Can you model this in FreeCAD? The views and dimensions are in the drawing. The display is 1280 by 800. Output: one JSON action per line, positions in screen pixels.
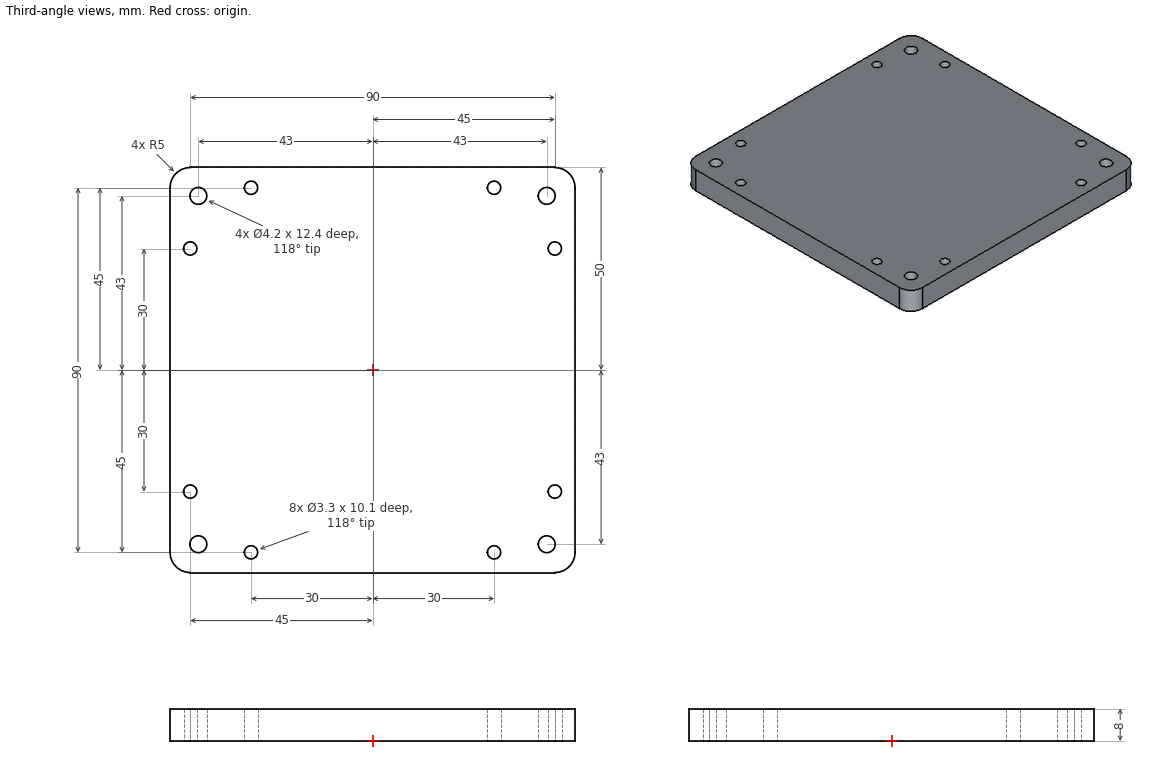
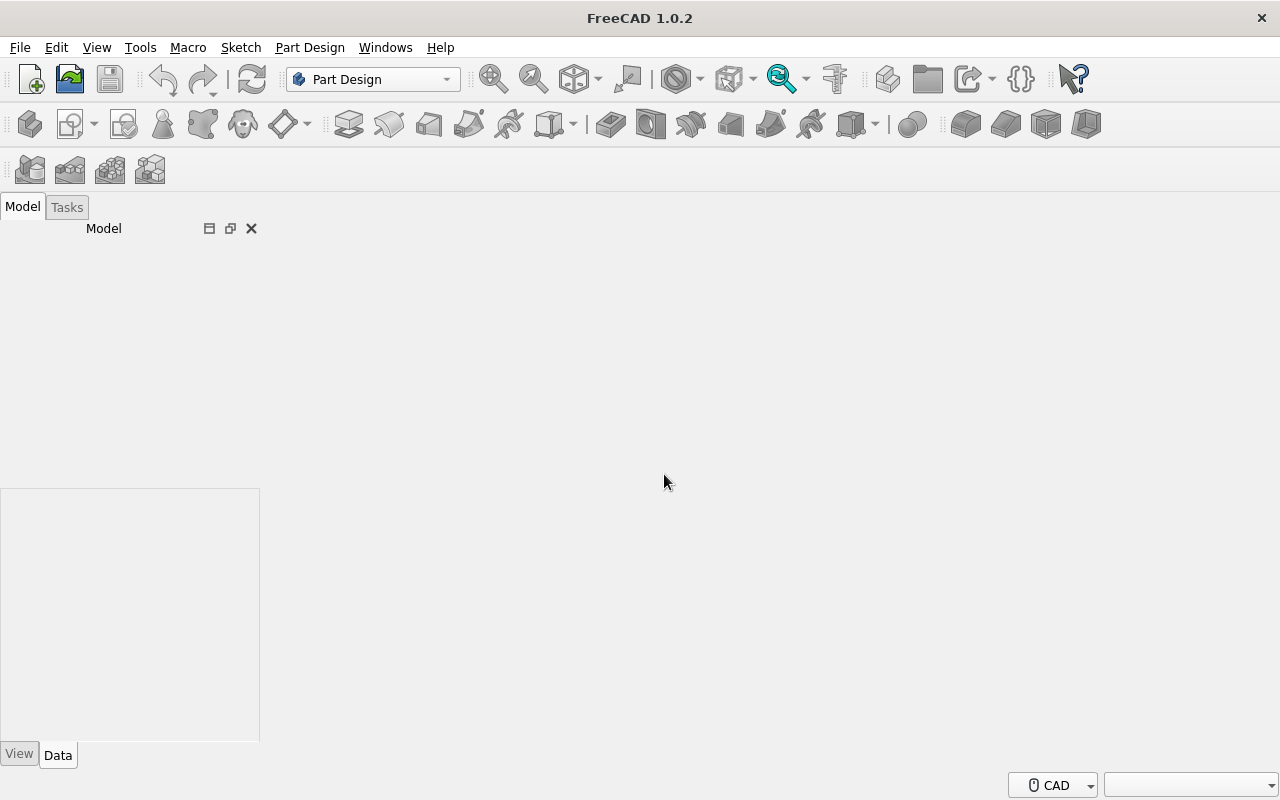
{"action": "left_click", "coordinate": [30, 80]}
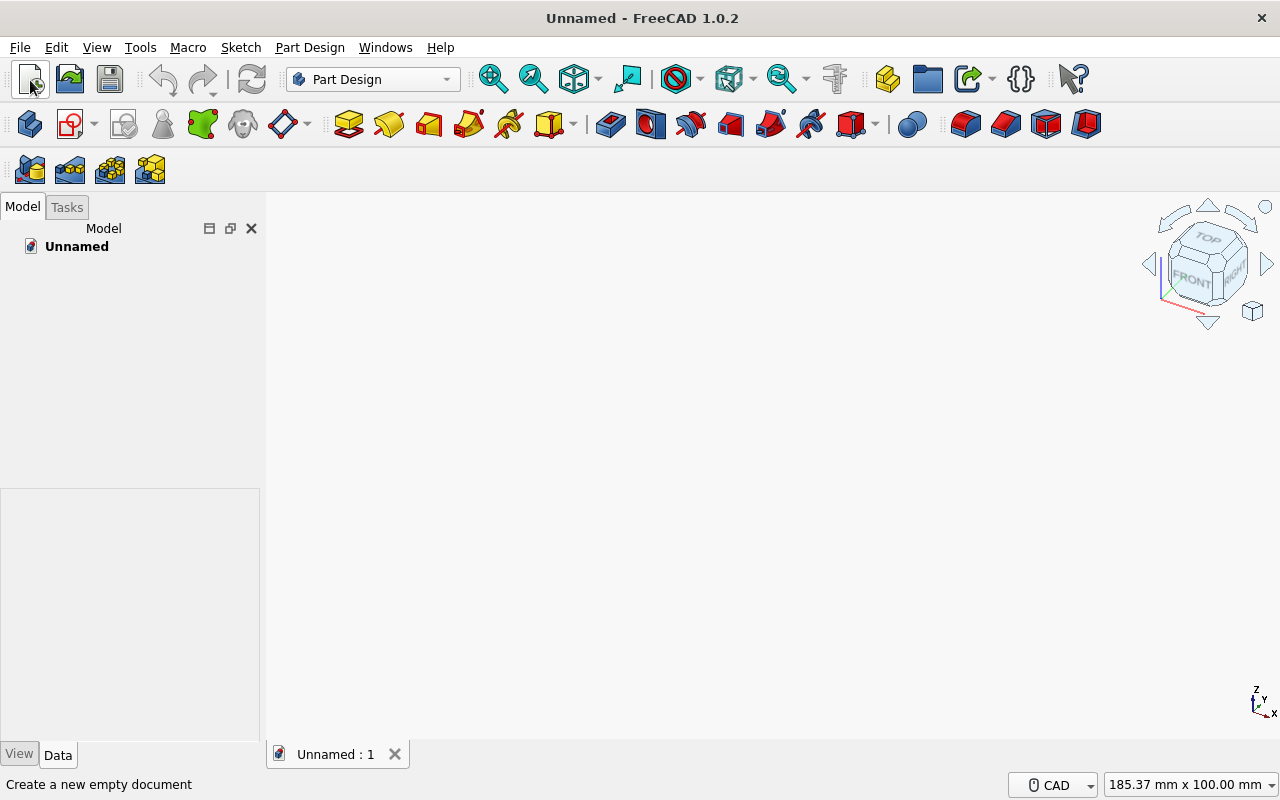
{"action": "left_click", "coordinate": [70, 124]}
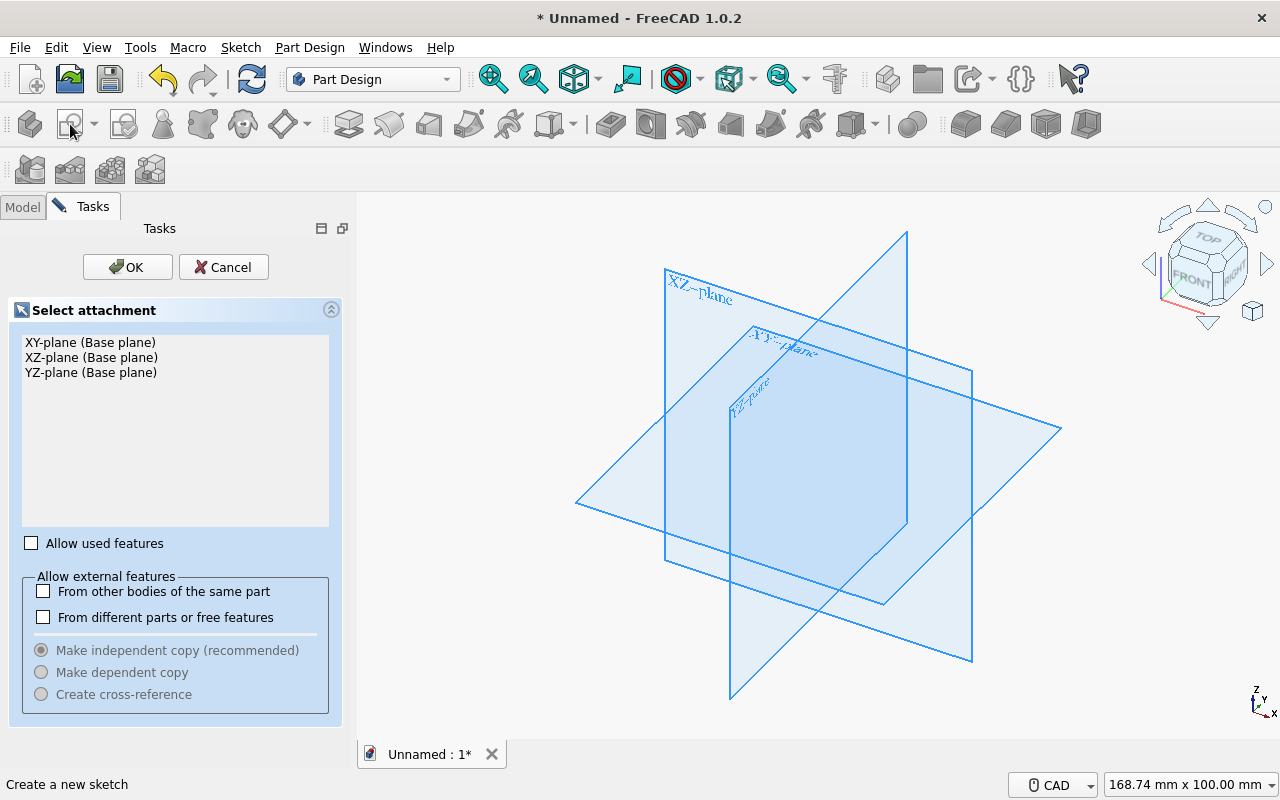
{"action": "left_click", "coordinate": [82, 342]}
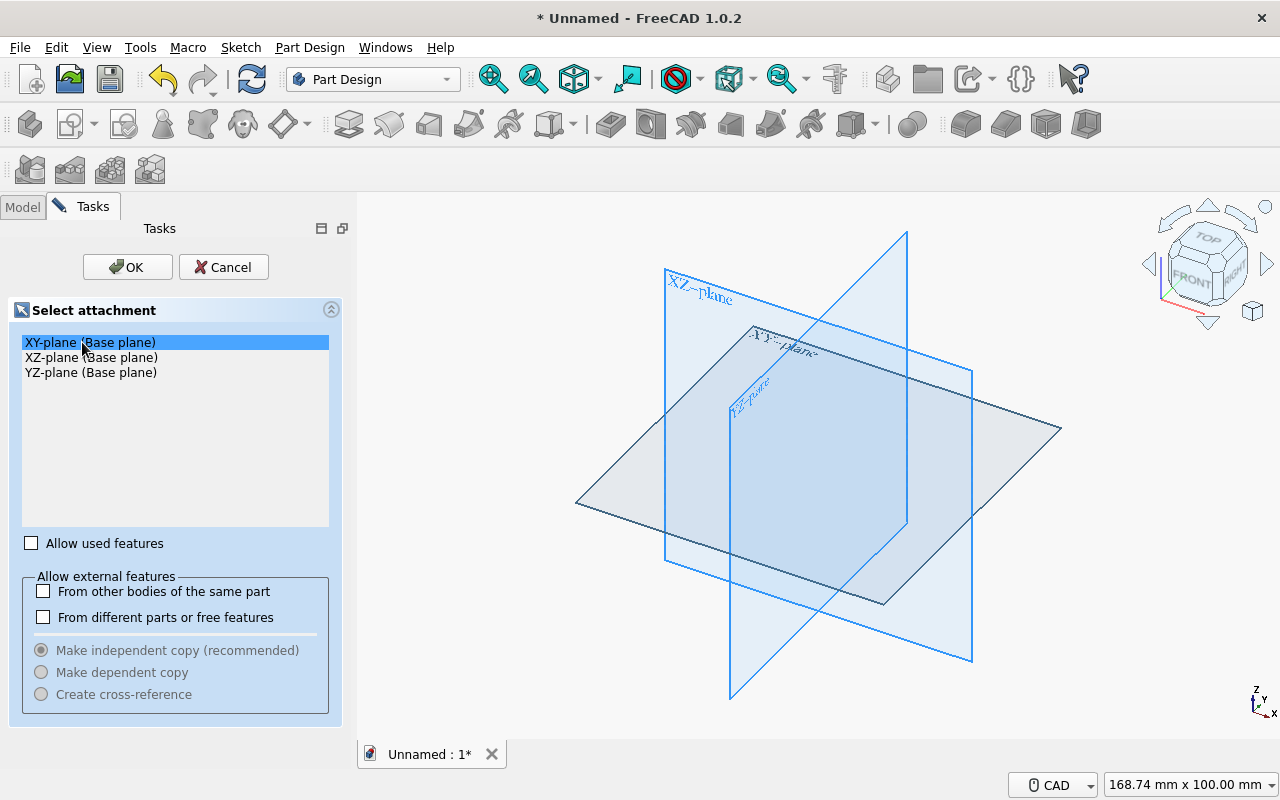
{"action": "left_click", "coordinate": [128, 267]}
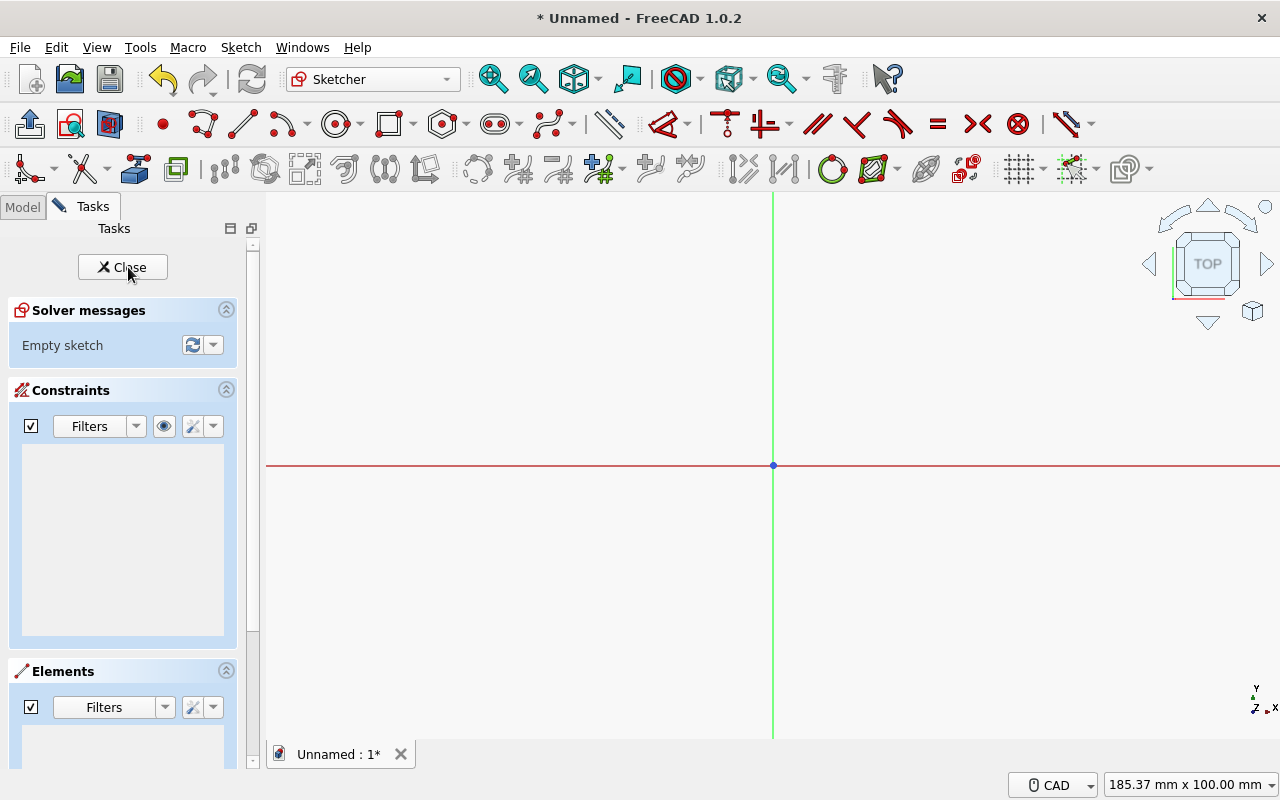
{"action": "scroll", "coordinate": [565, 466], "scroll_direction": "down", "scroll_amount": 2}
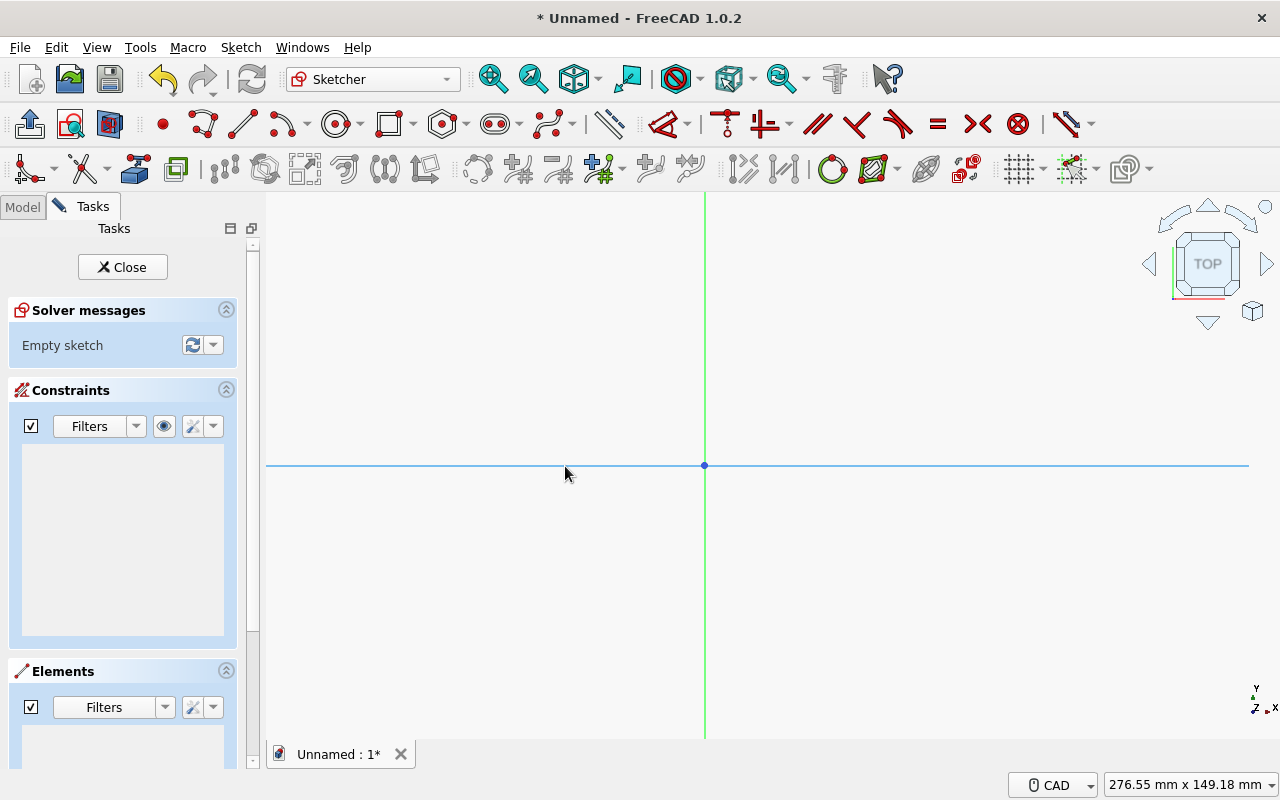
{"action": "left_click", "coordinate": [244, 124]}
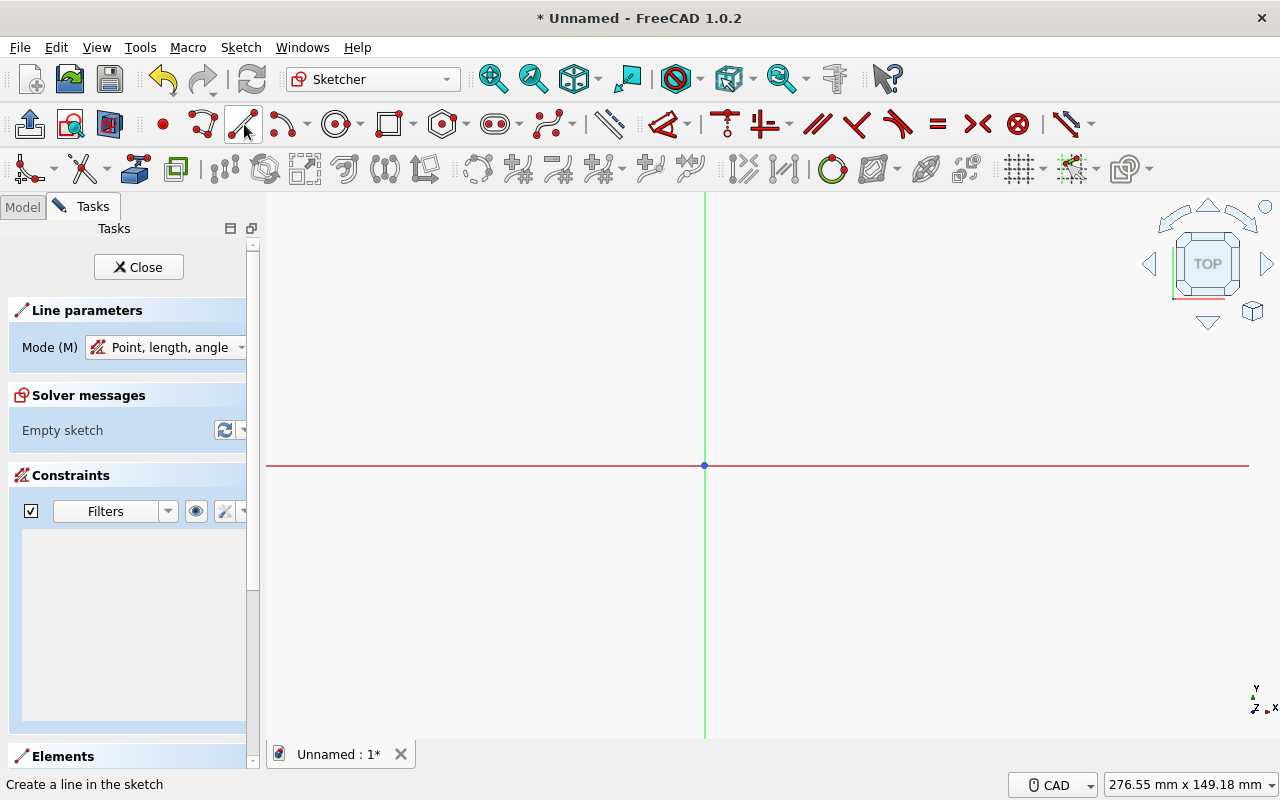
{"action": "left_click", "coordinate": [870, 282]}
{"action": "left_click", "coordinate": [540, 282]}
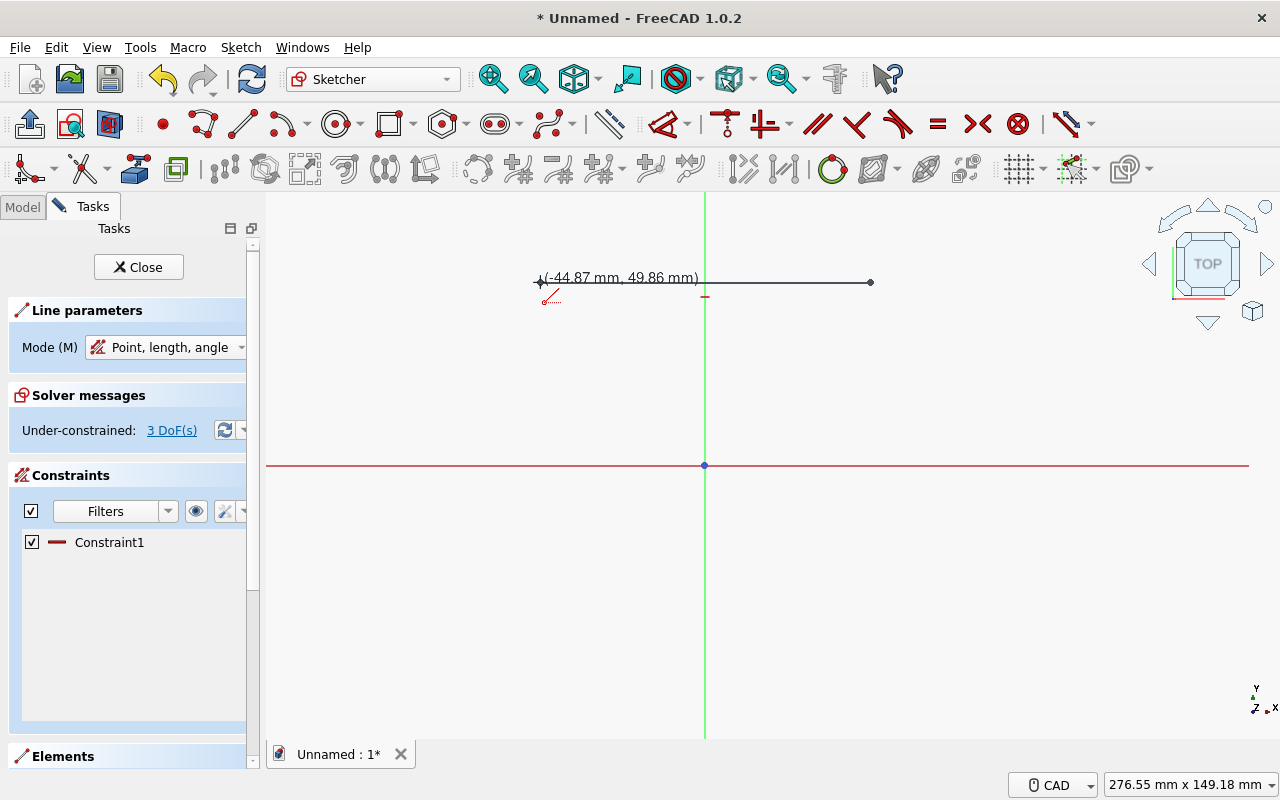
{"action": "left_click", "coordinate": [521, 301]}
{"action": "left_click", "coordinate": [521, 631]}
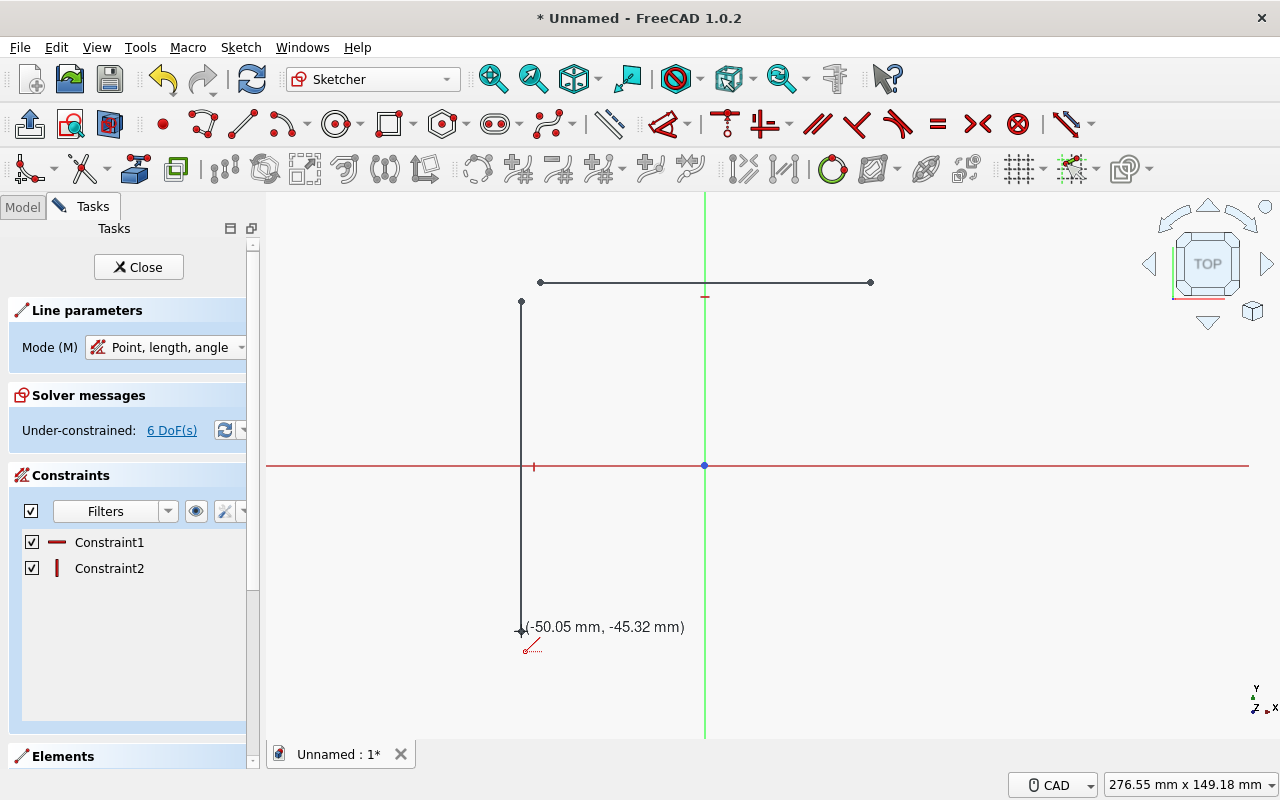
{"action": "left_click", "coordinate": [540, 649]}
{"action": "left_click", "coordinate": [870, 649]}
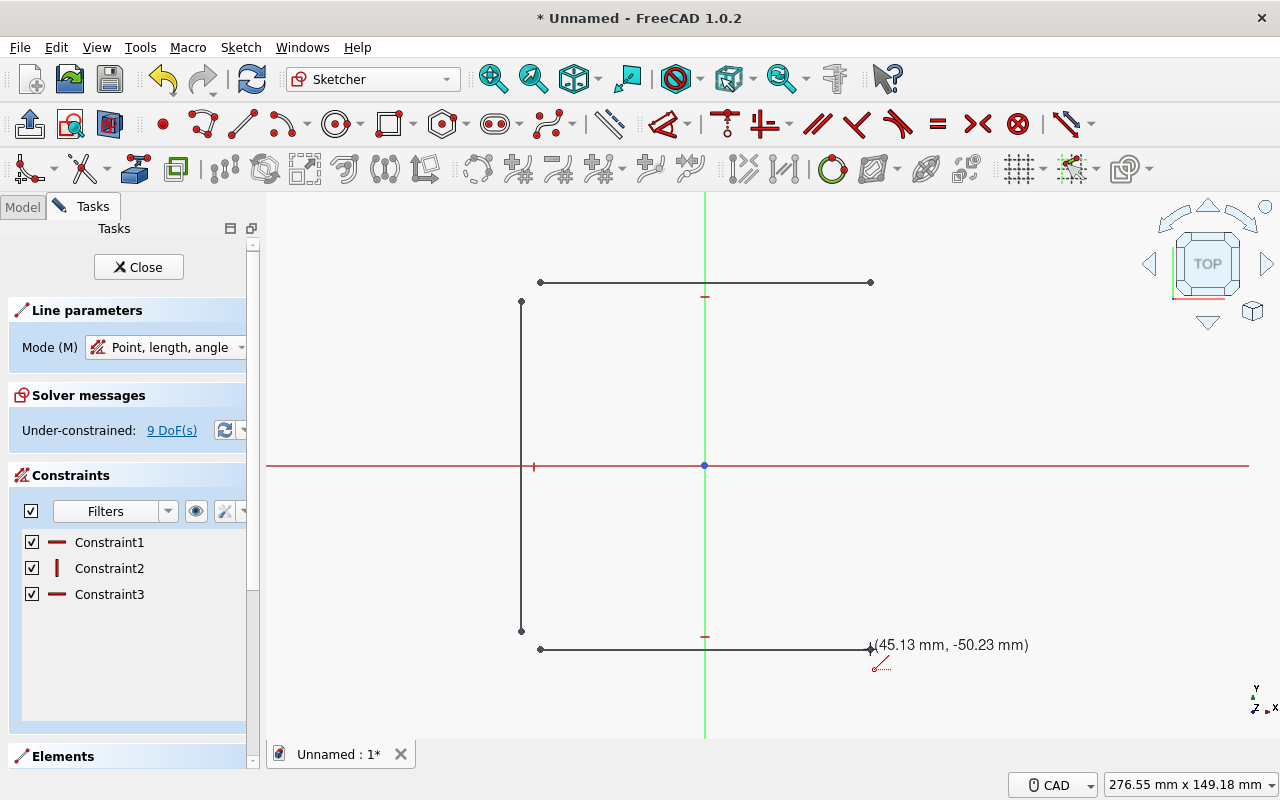
{"action": "left_click", "coordinate": [888, 631]}
{"action": "left_click", "coordinate": [888, 301]}